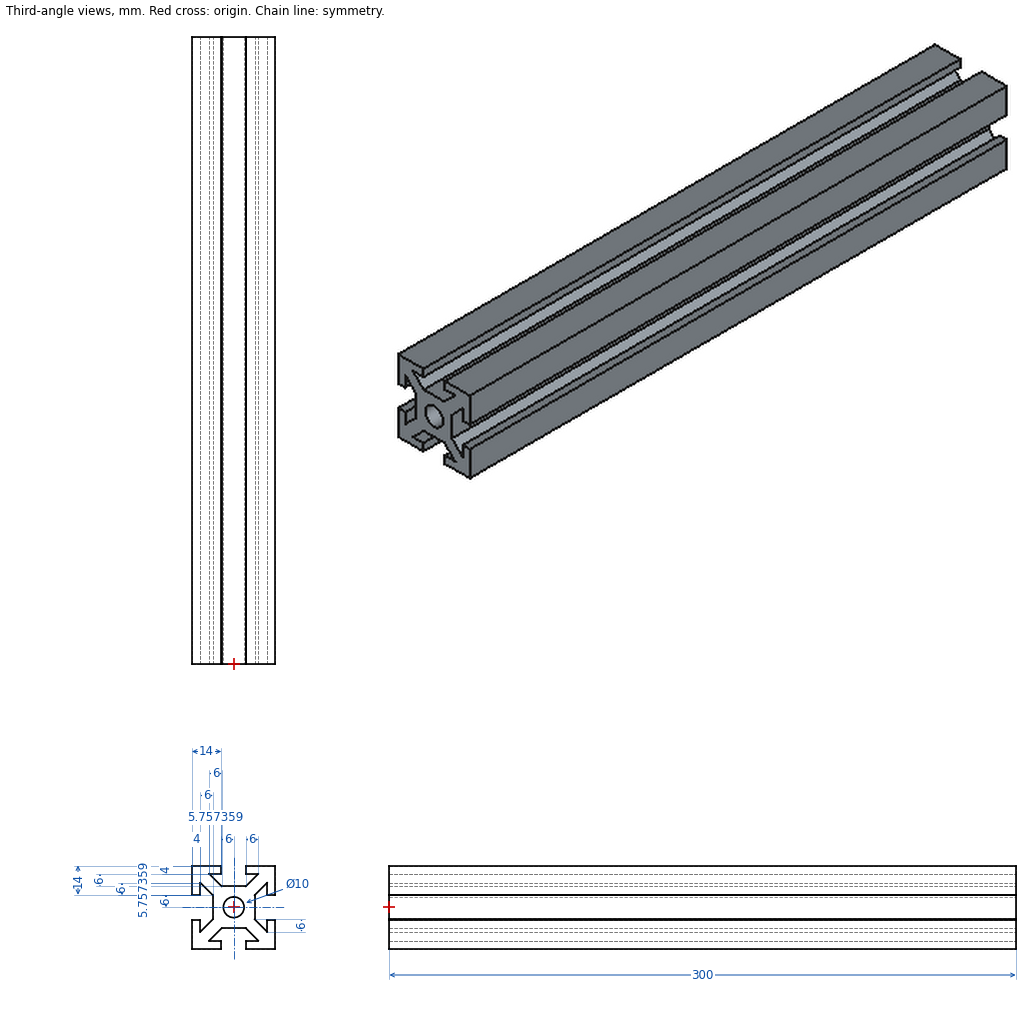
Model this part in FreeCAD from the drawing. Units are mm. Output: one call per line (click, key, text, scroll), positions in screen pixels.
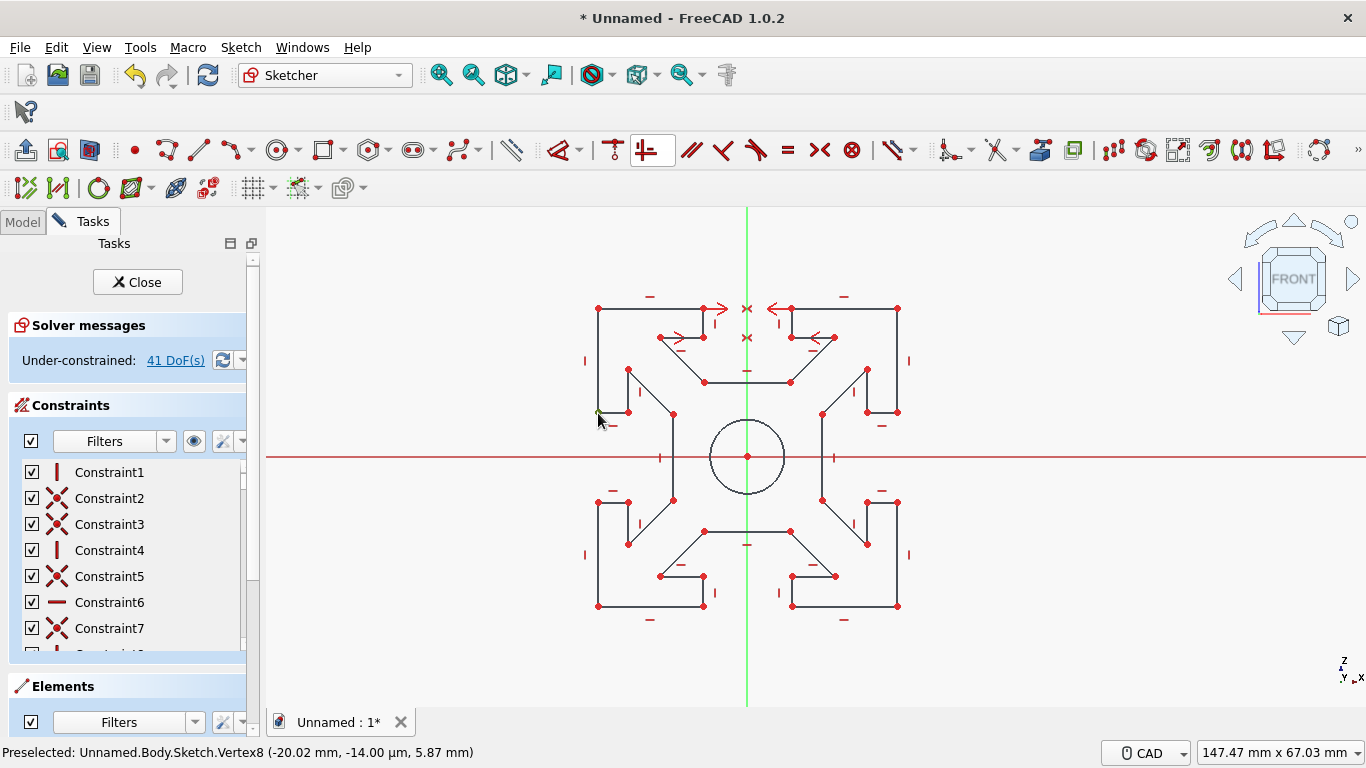
click(897, 413)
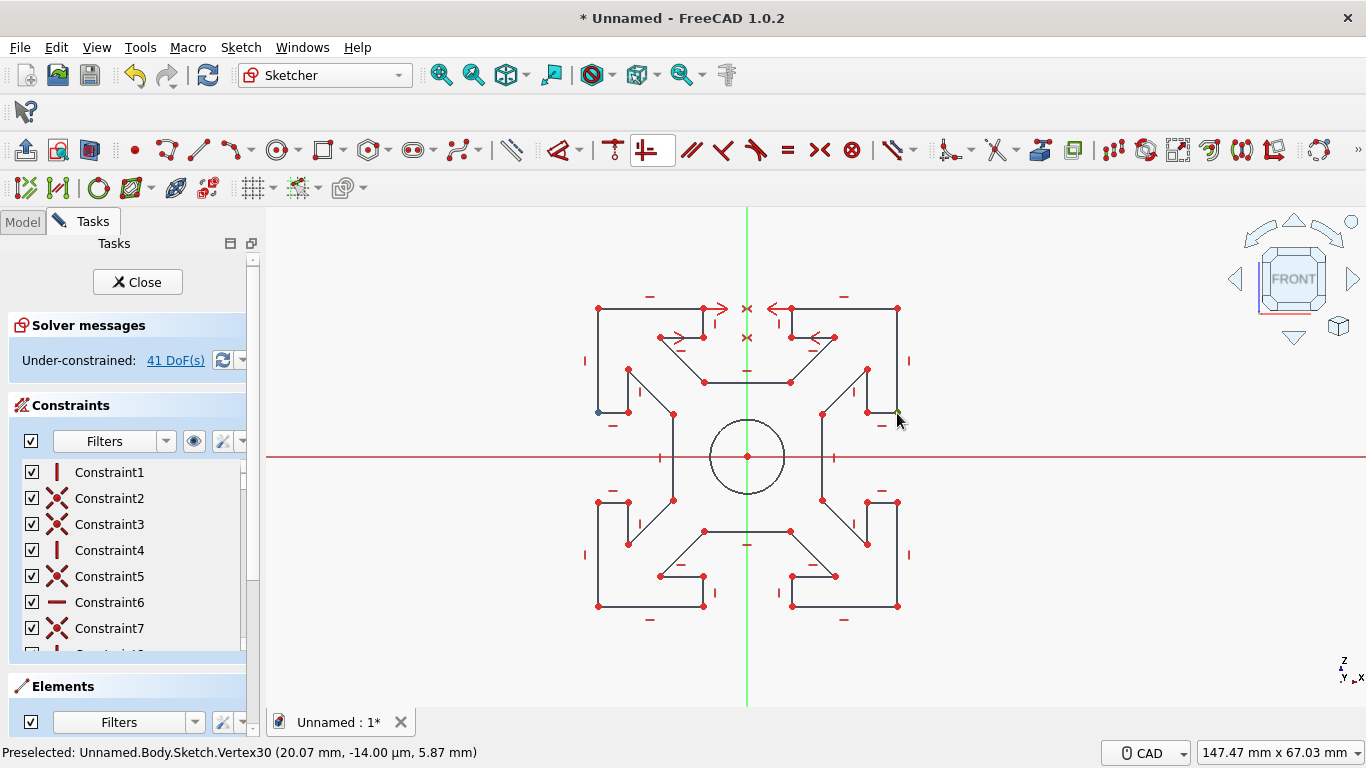
click(747, 647)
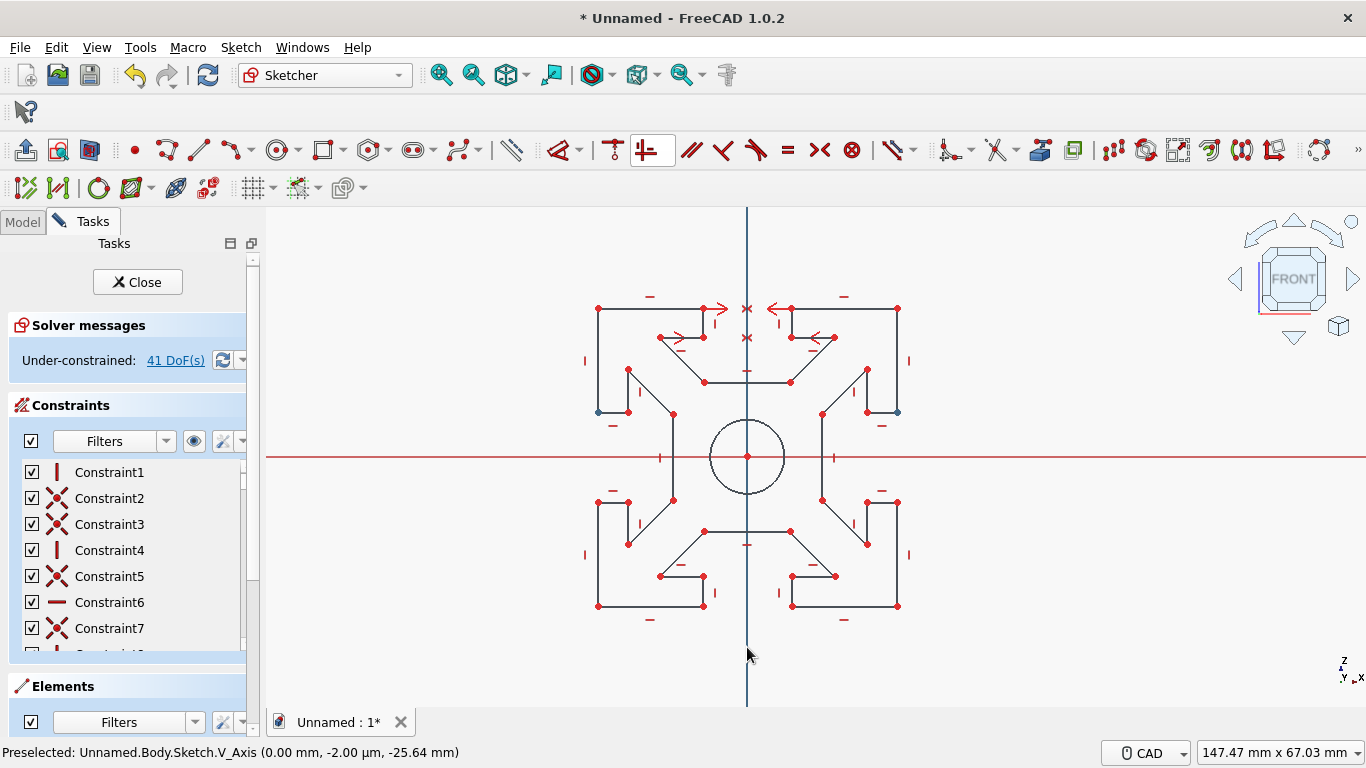
click(820, 150)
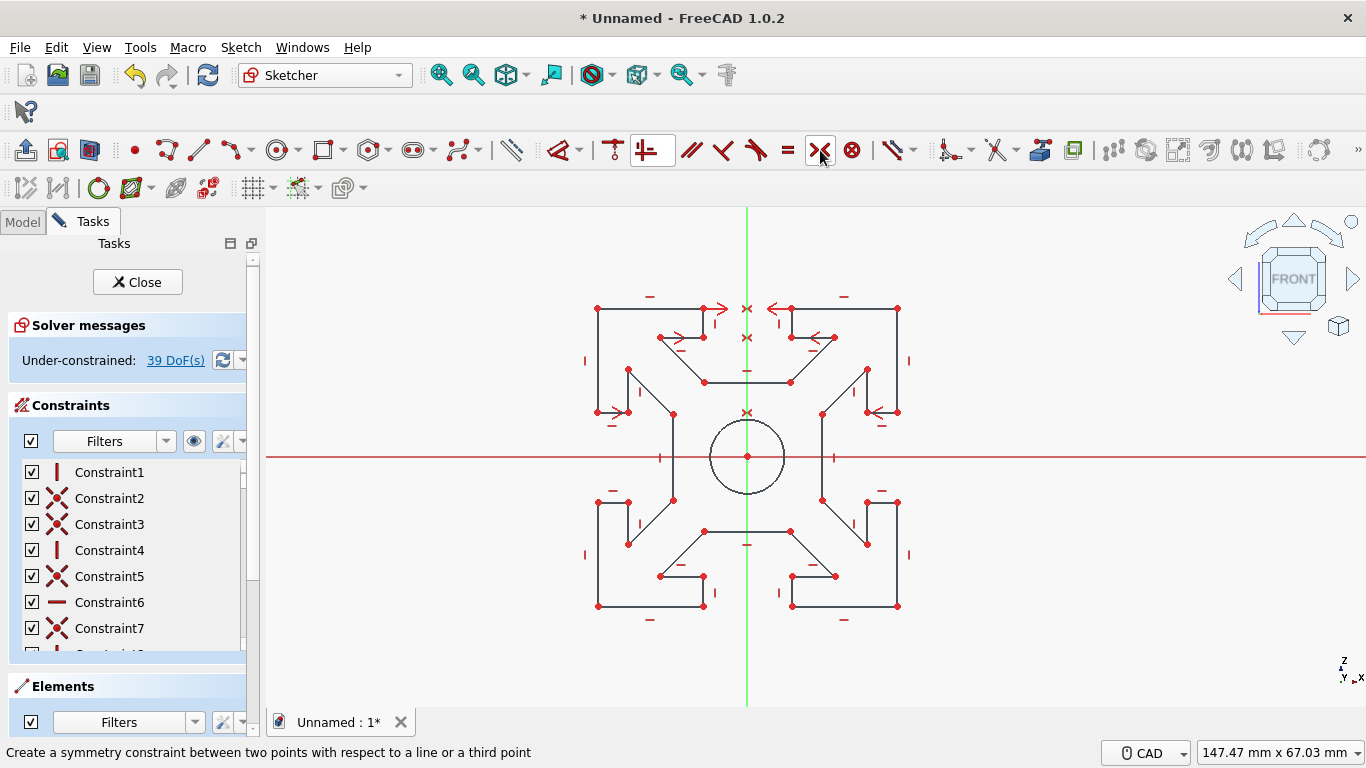
click(628, 370)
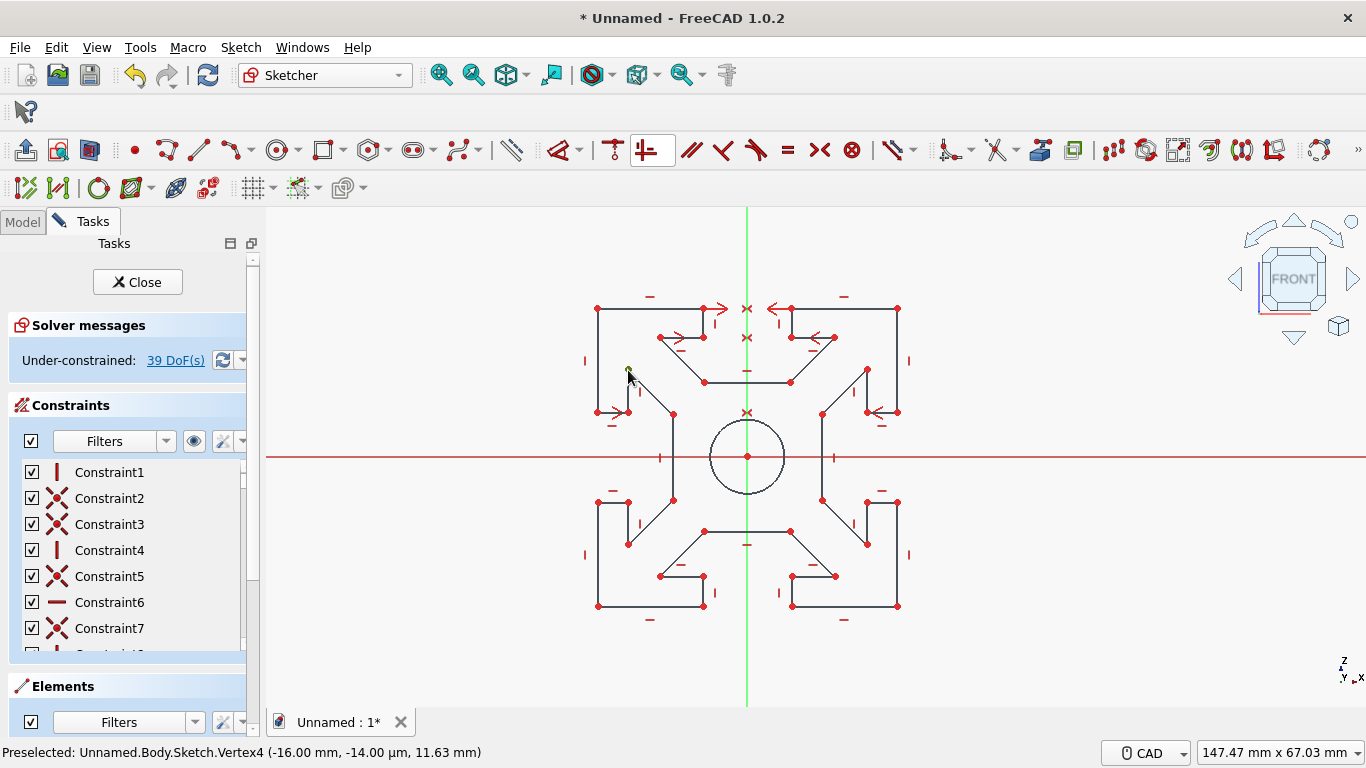
click(867, 370)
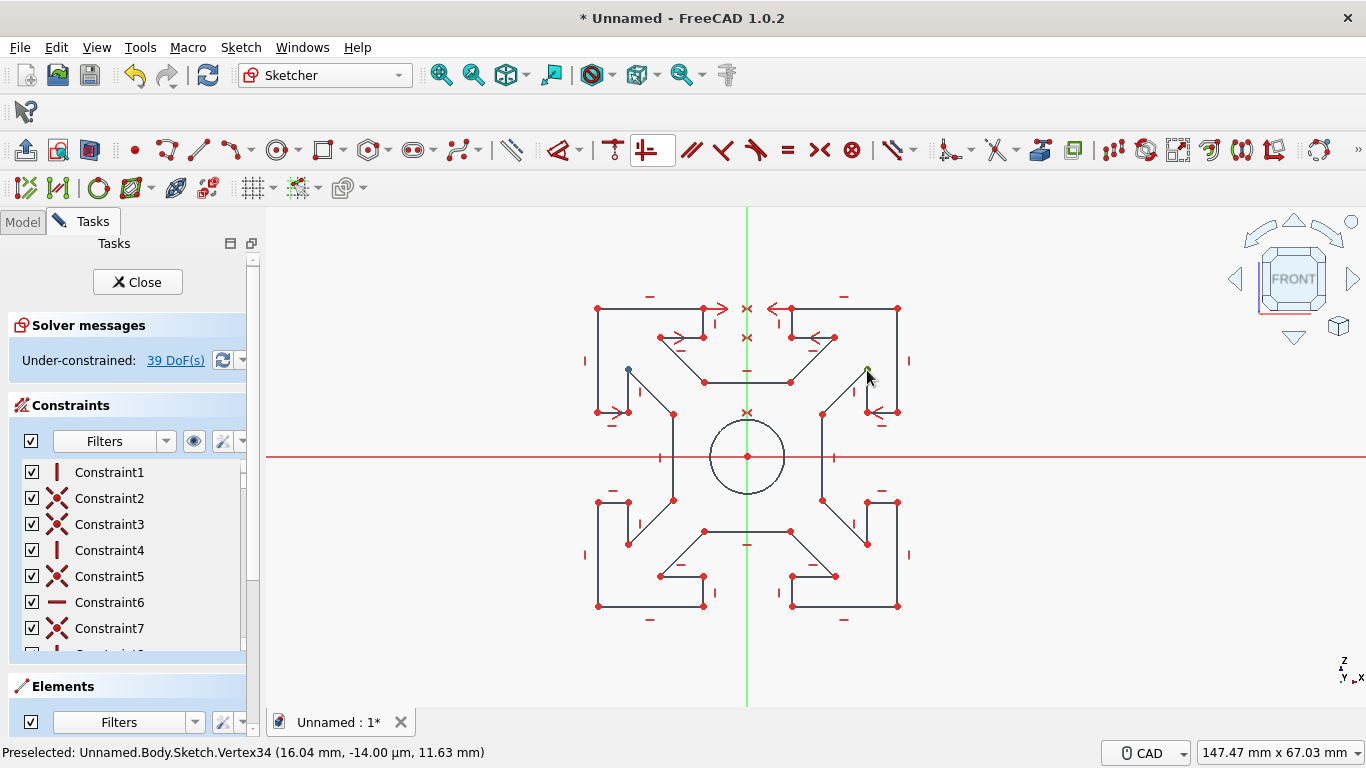
click(747, 647)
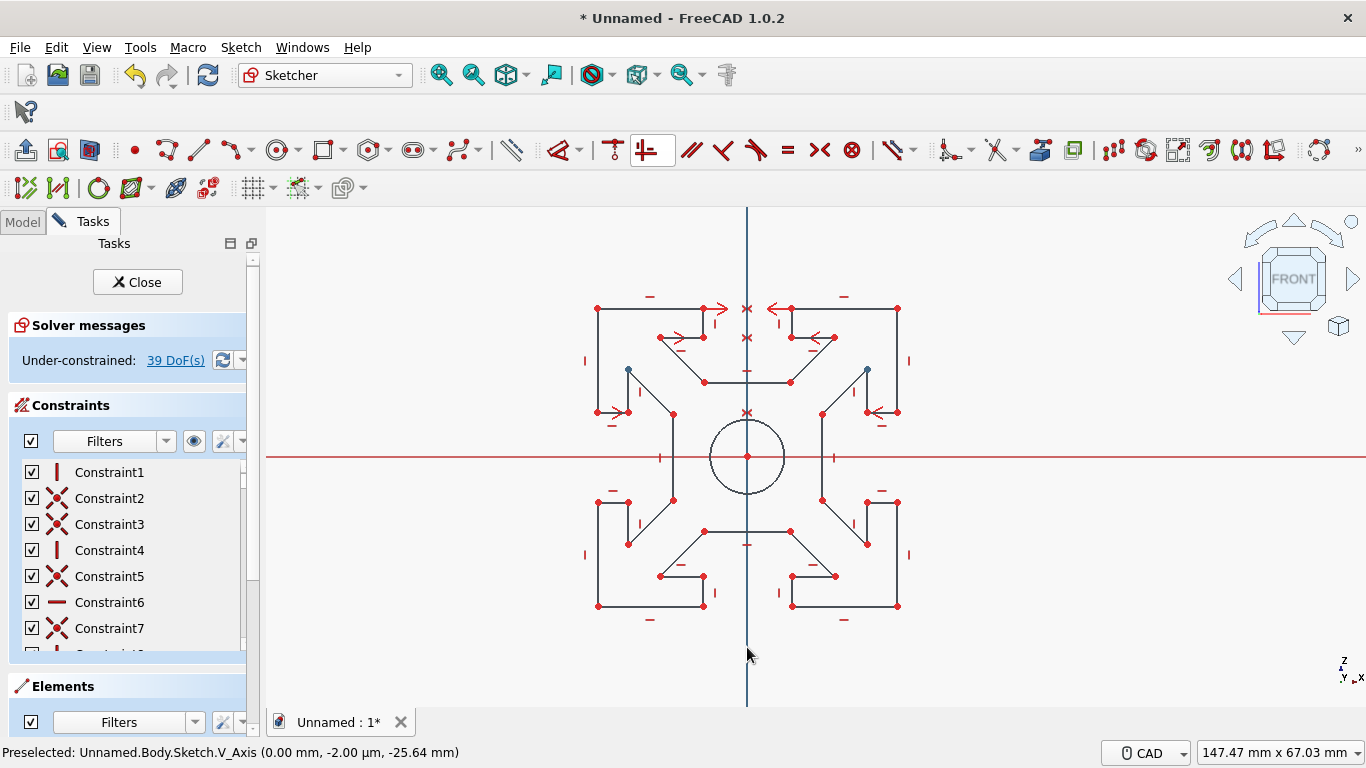
click(820, 150)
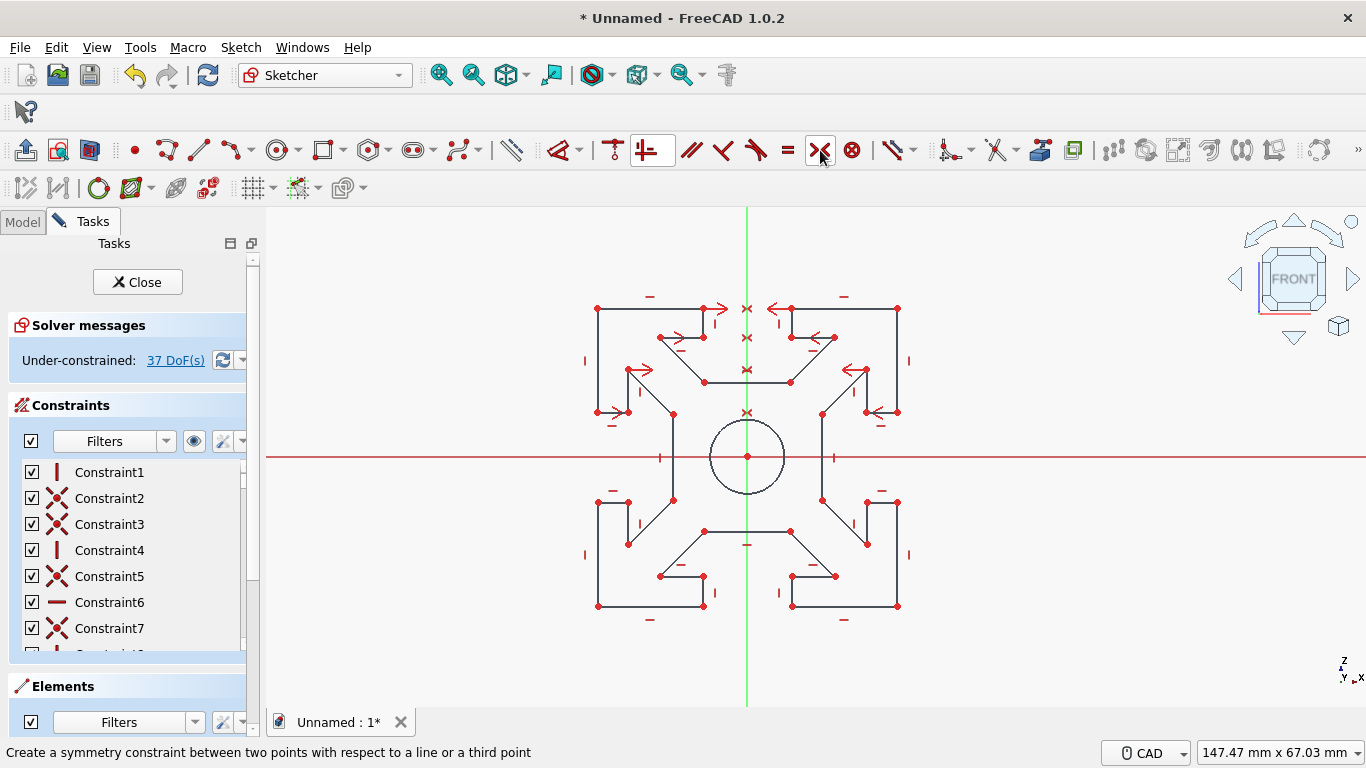
click(673, 415)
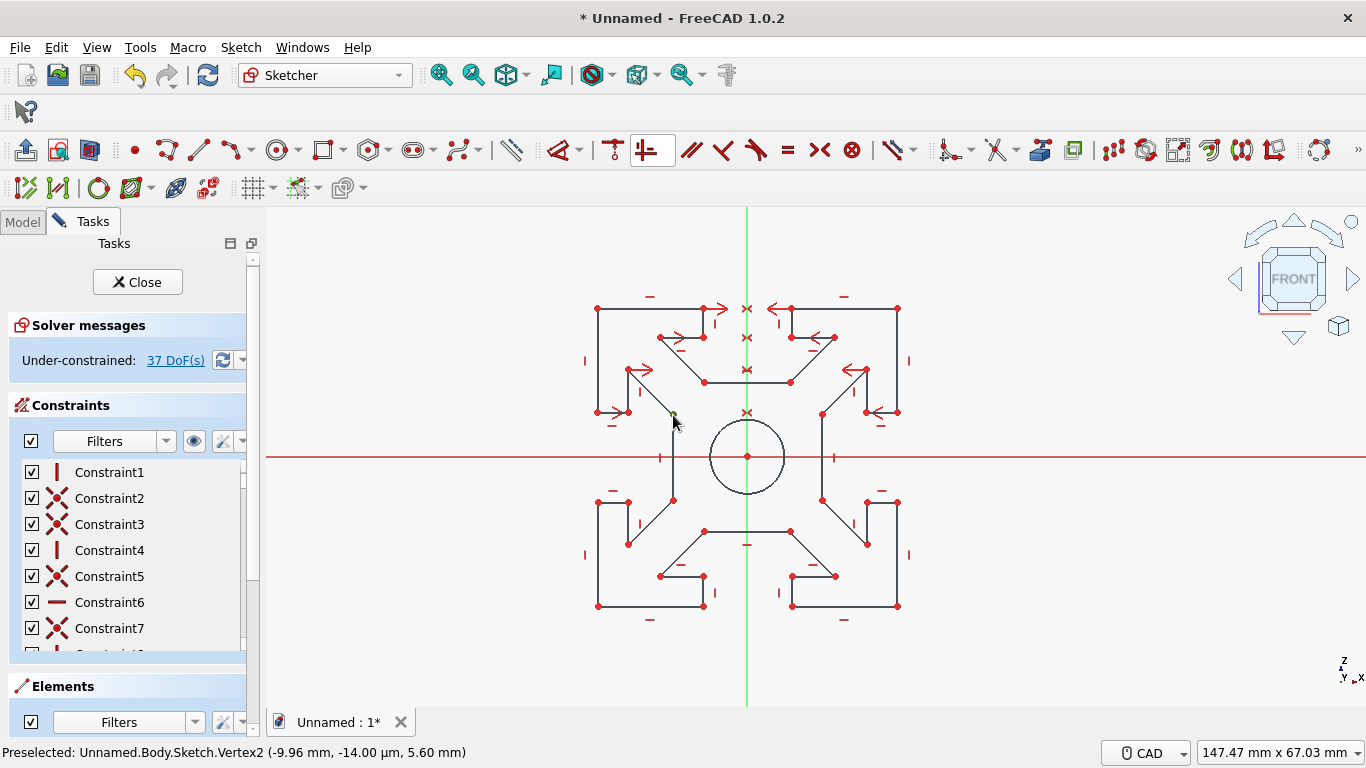
click(822, 415)